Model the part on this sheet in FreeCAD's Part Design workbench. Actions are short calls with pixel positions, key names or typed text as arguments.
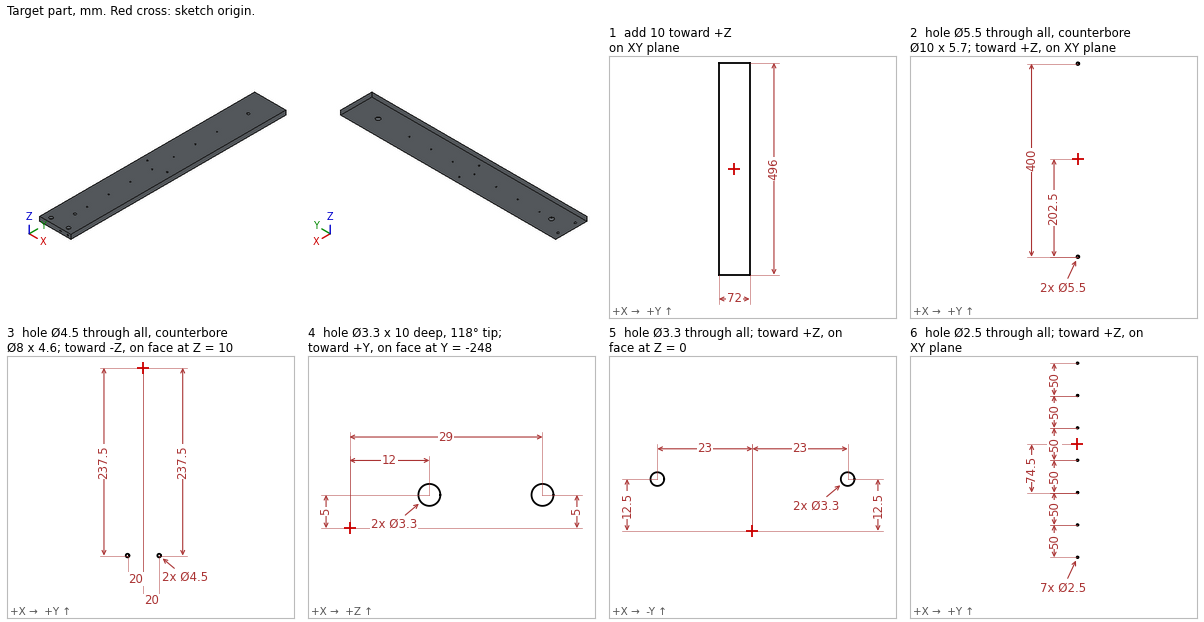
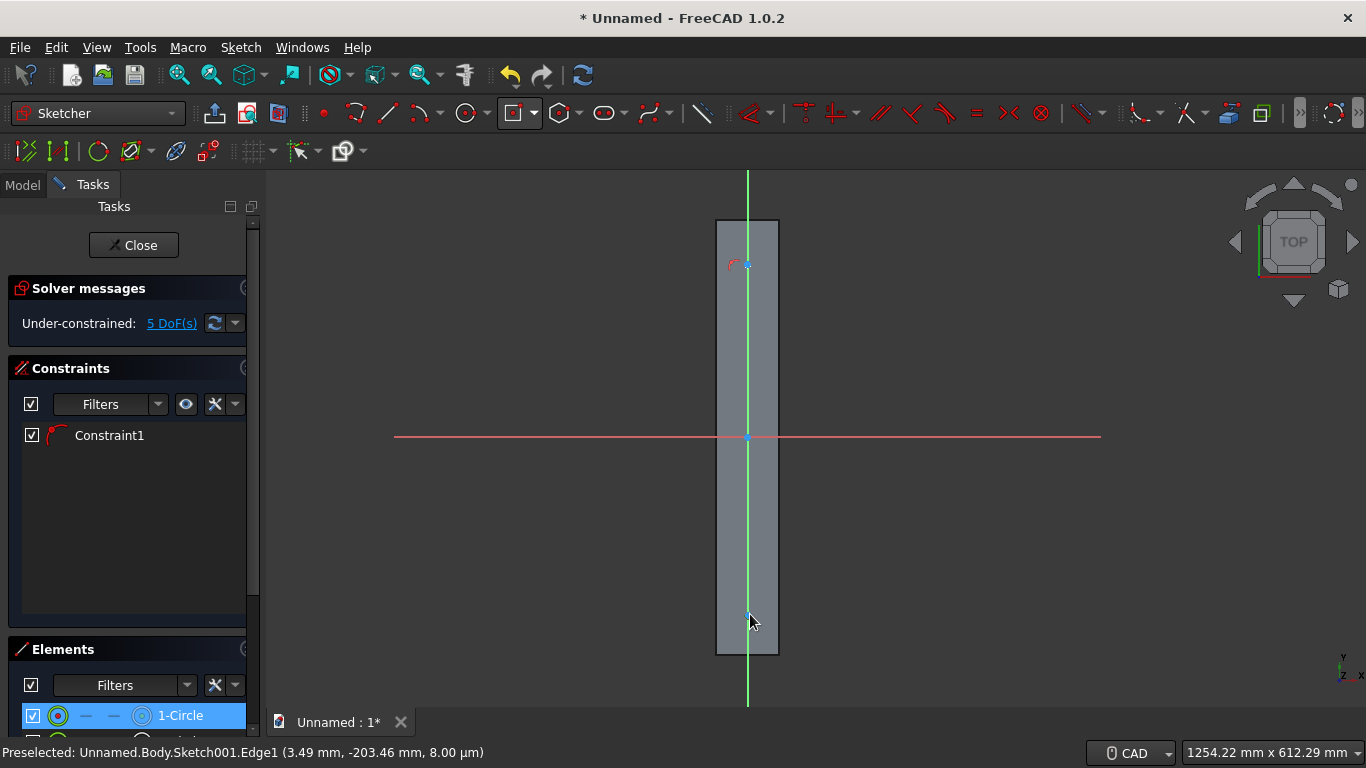
scroll(749, 263, up, 10)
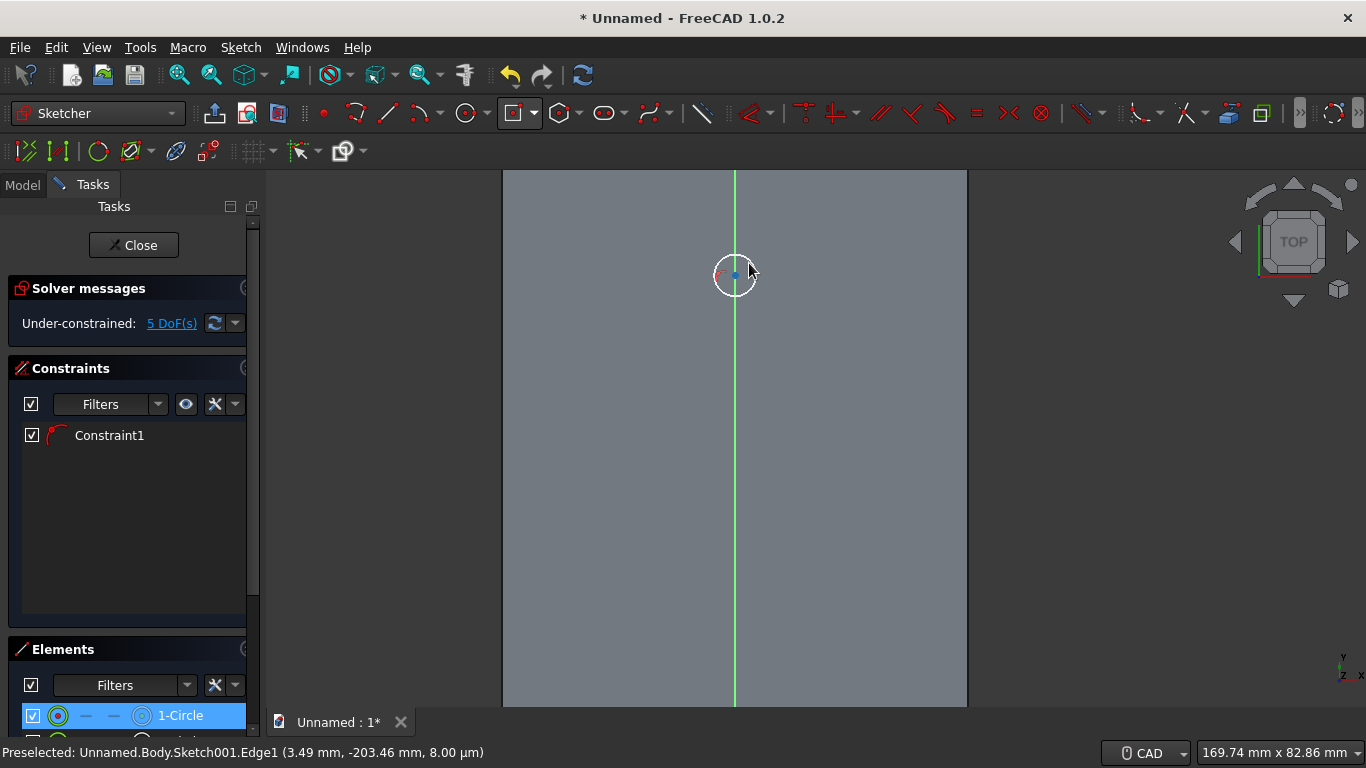
click(750, 261)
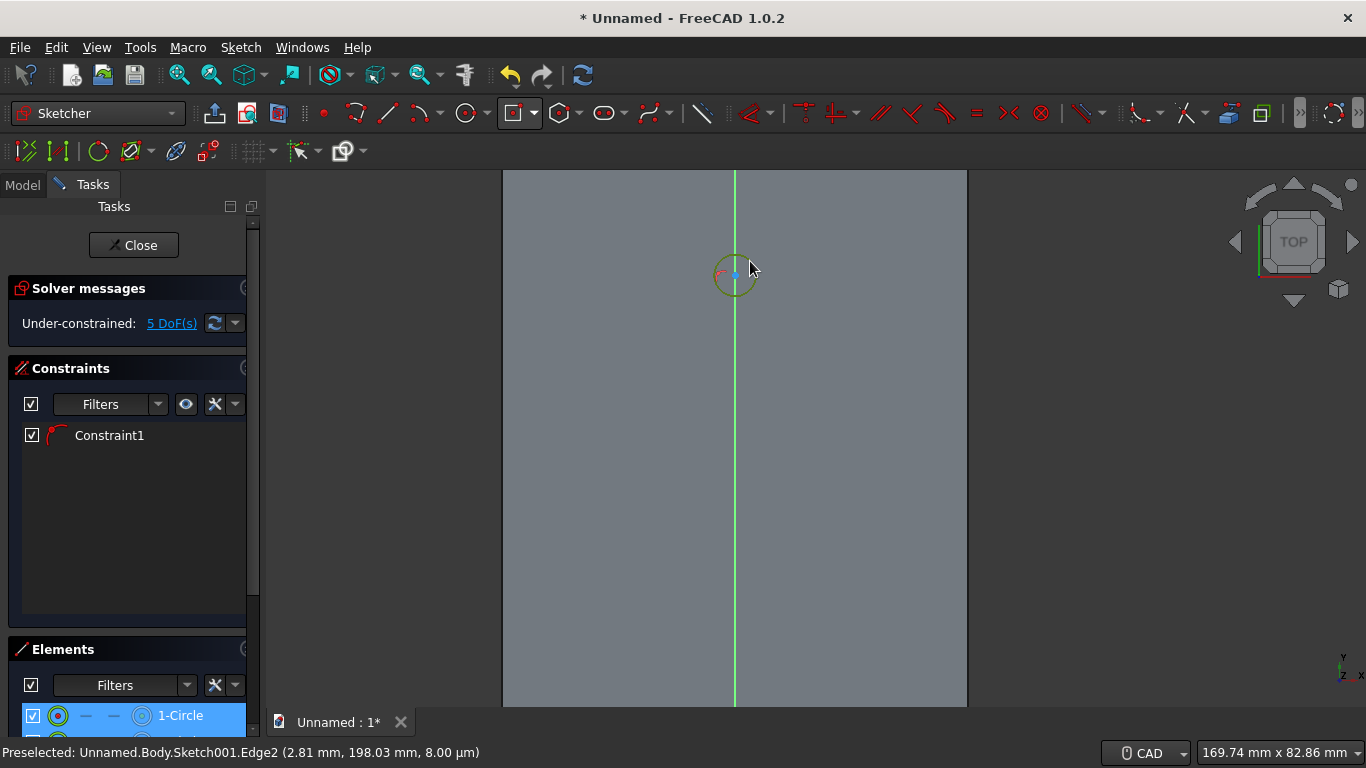
click(978, 114)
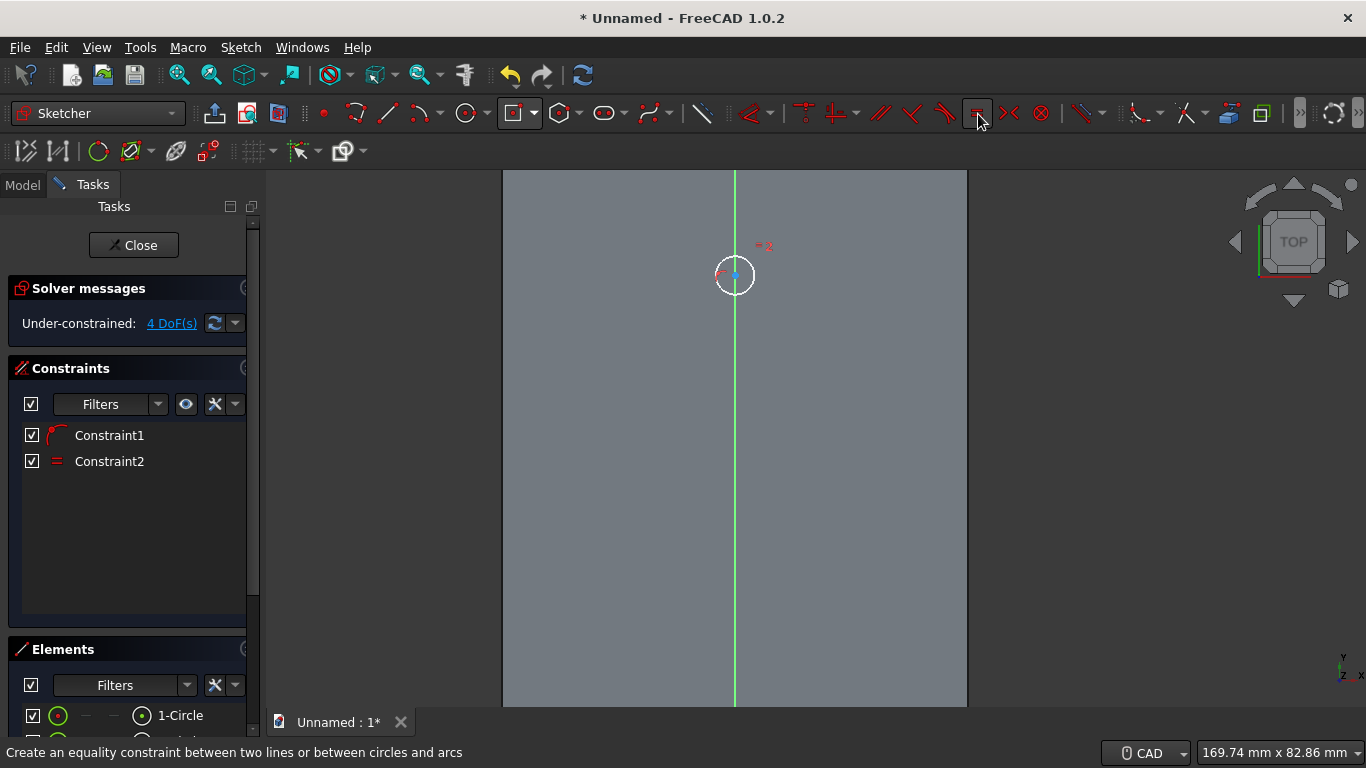
scroll(749, 262, down, 10)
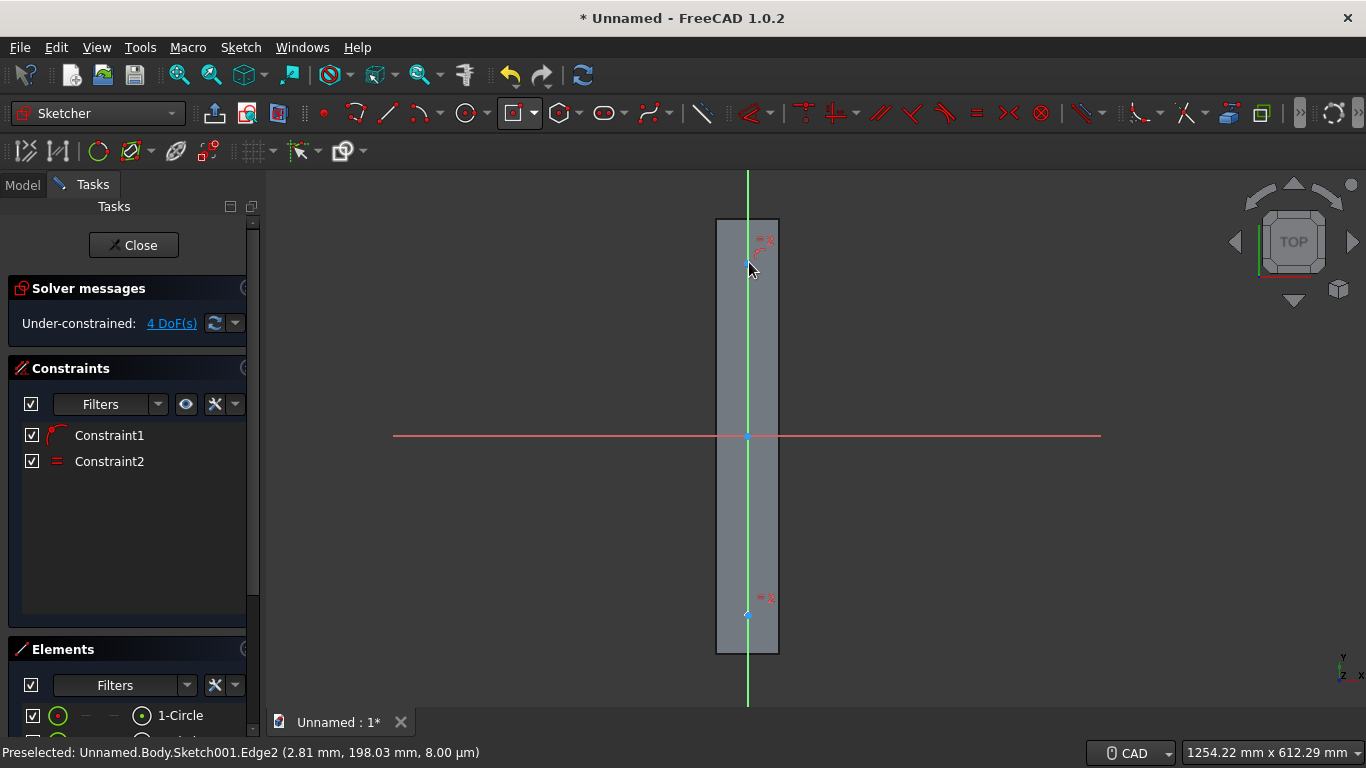
click(748, 615)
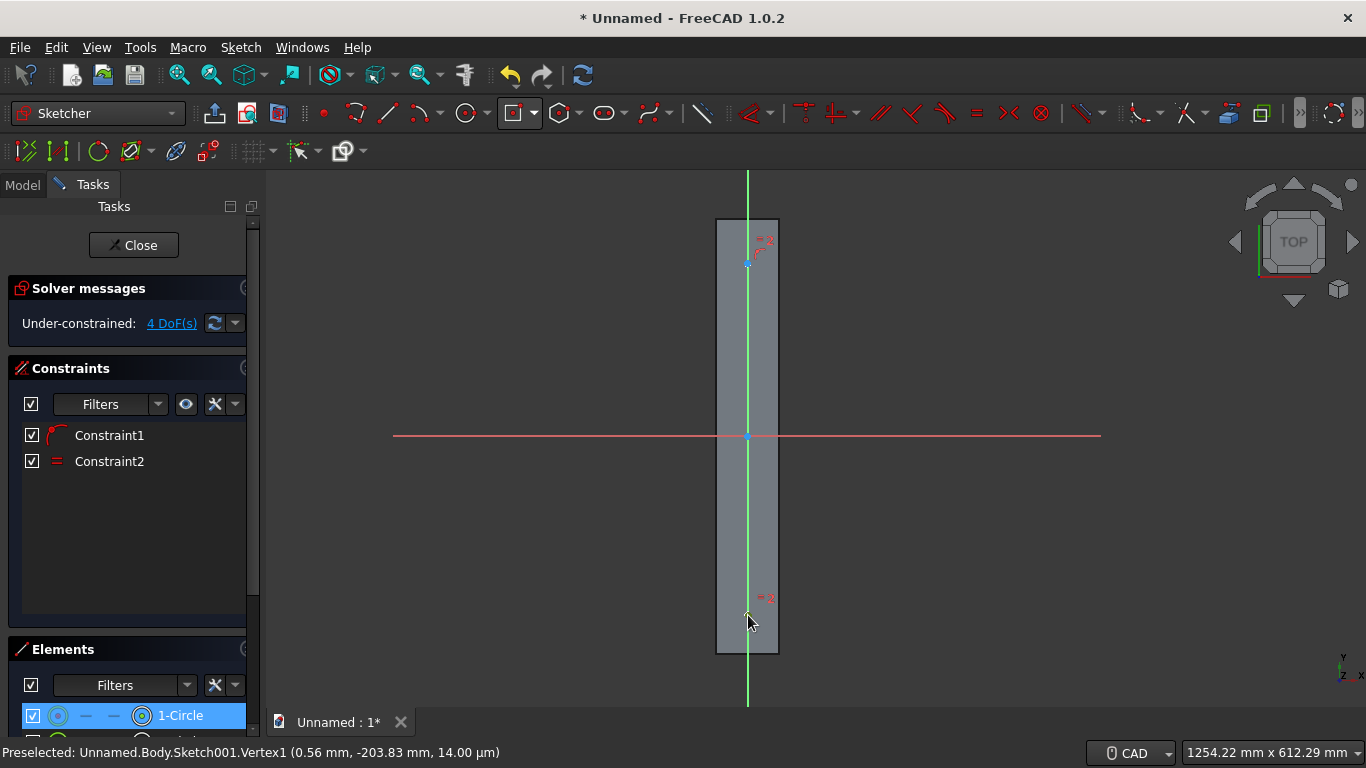
click(748, 576)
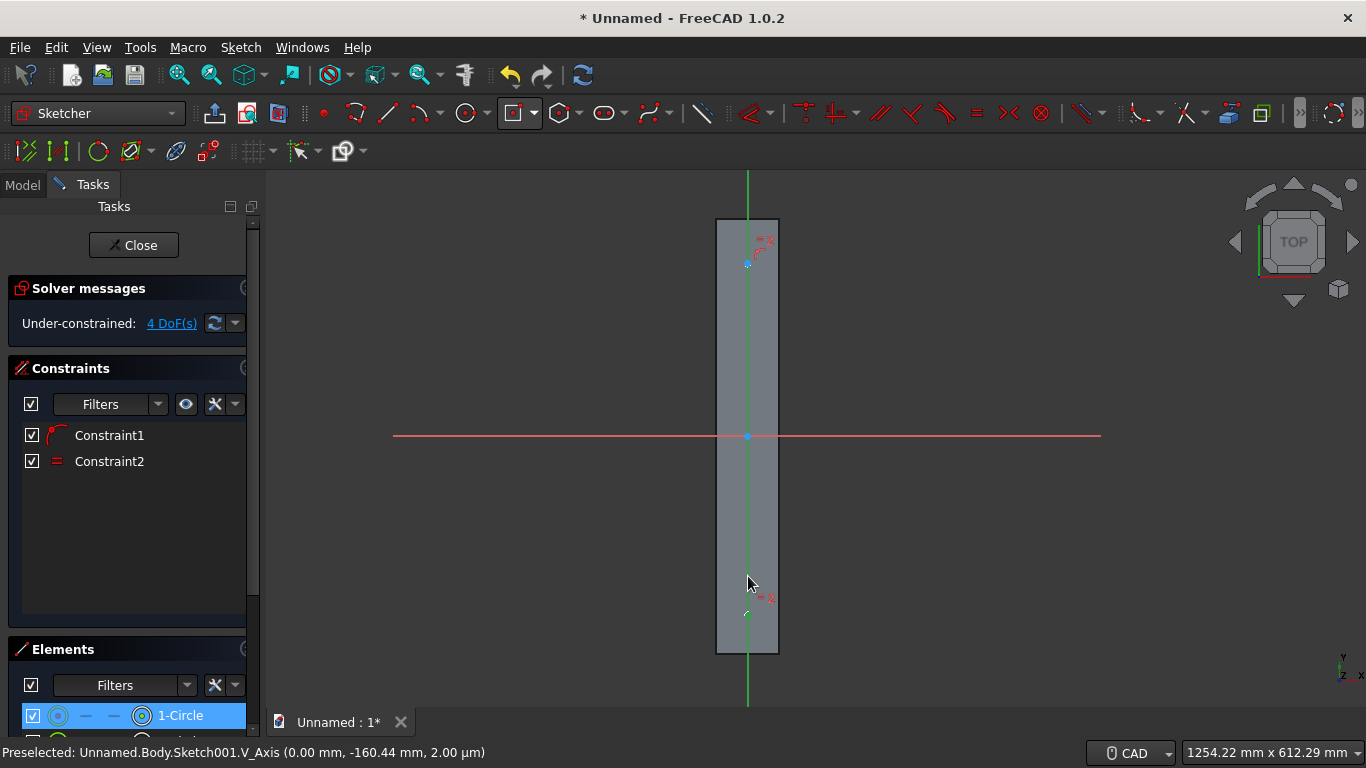
click(804, 114)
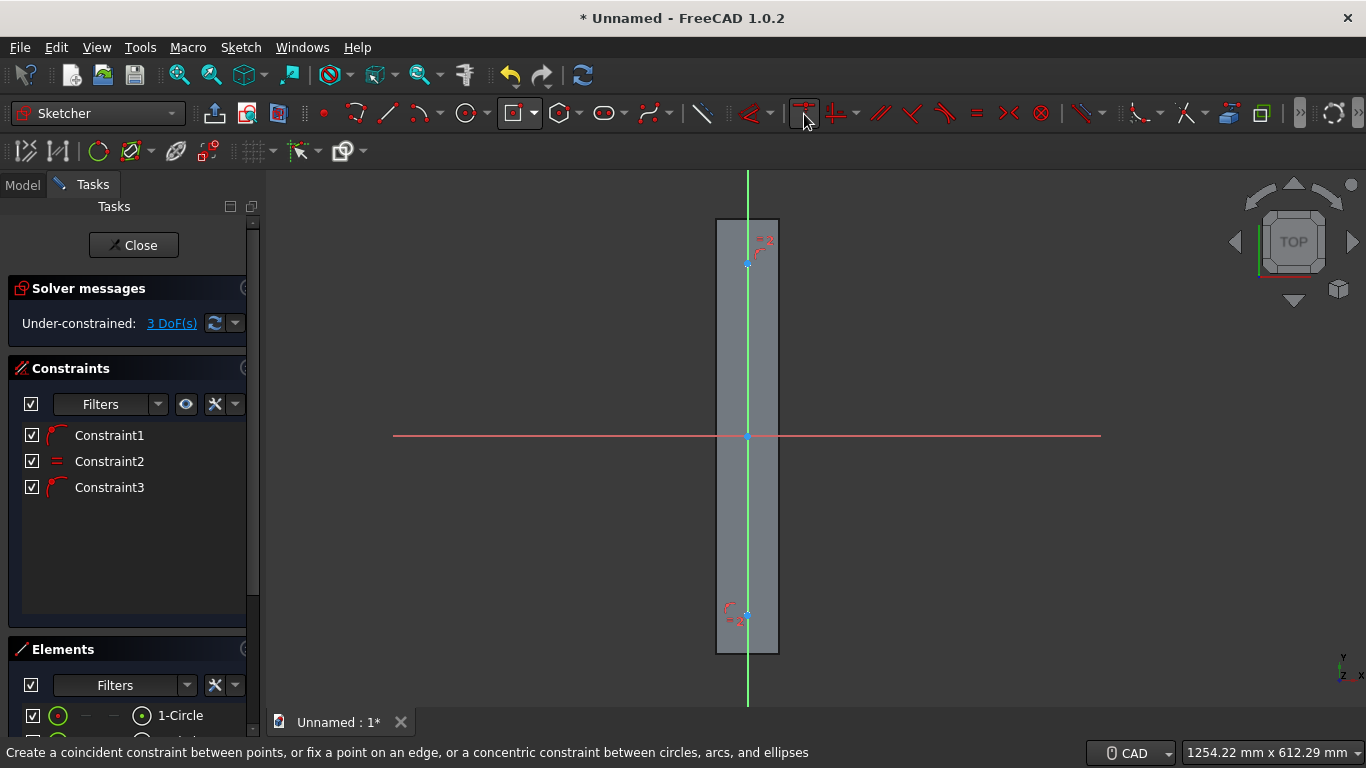
click(750, 114)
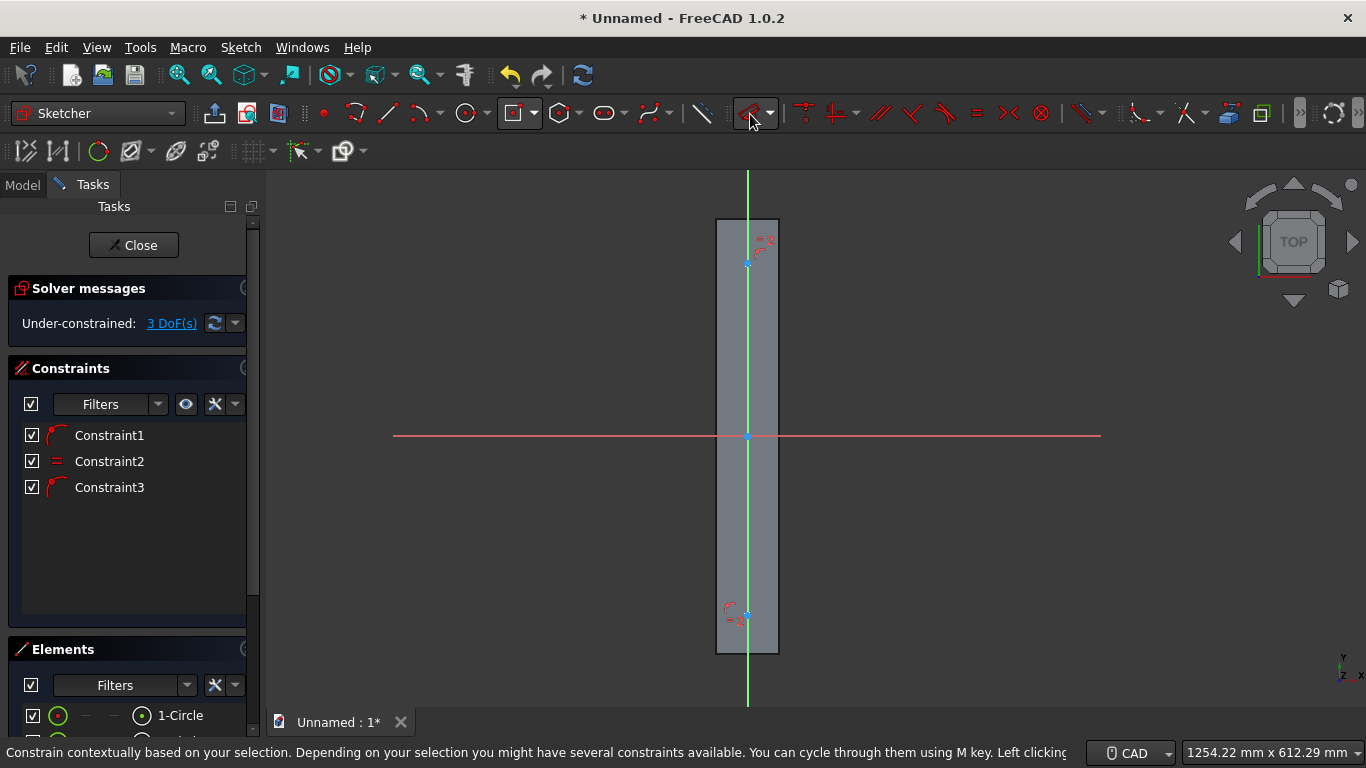
scroll(749, 613, up, 11)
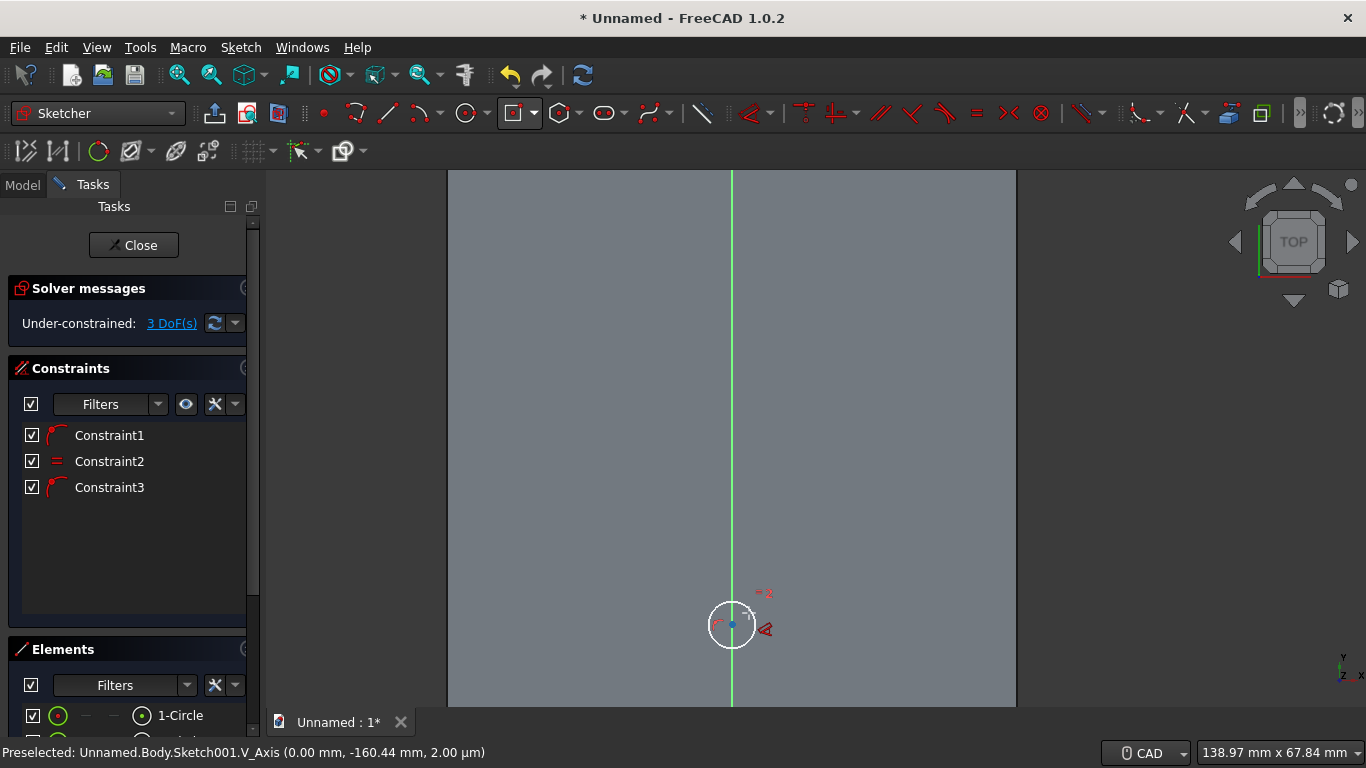
click(748, 608)
click(770, 585)